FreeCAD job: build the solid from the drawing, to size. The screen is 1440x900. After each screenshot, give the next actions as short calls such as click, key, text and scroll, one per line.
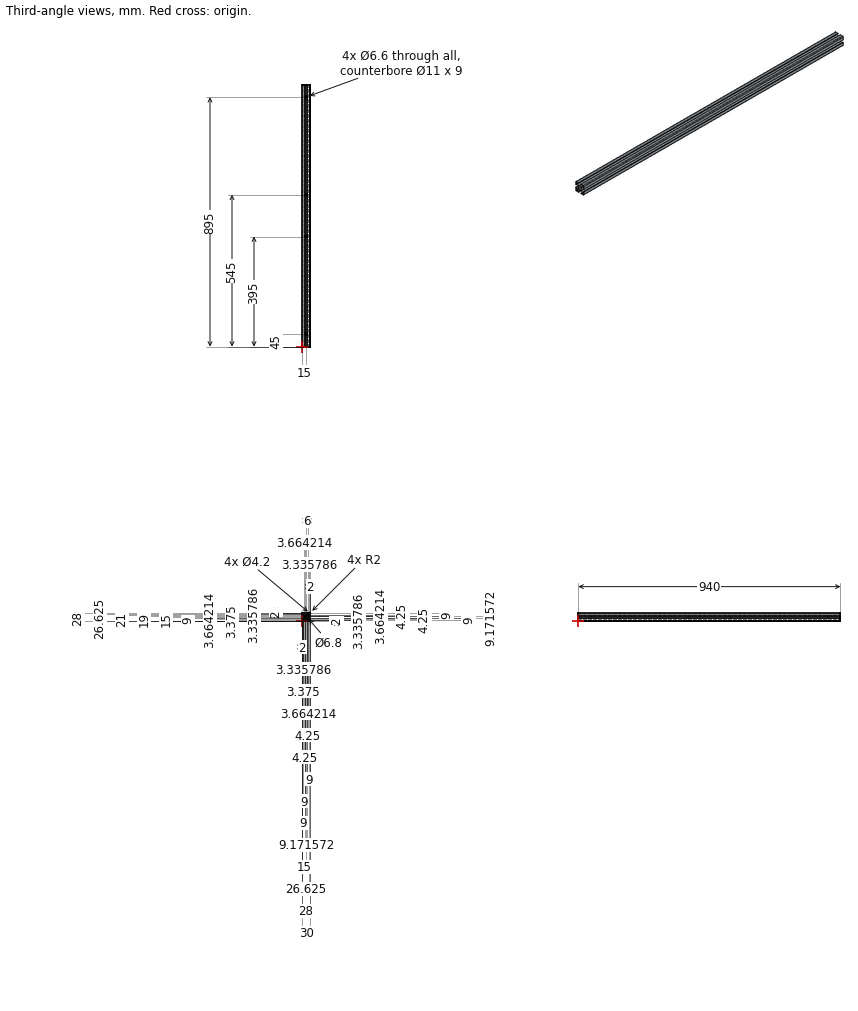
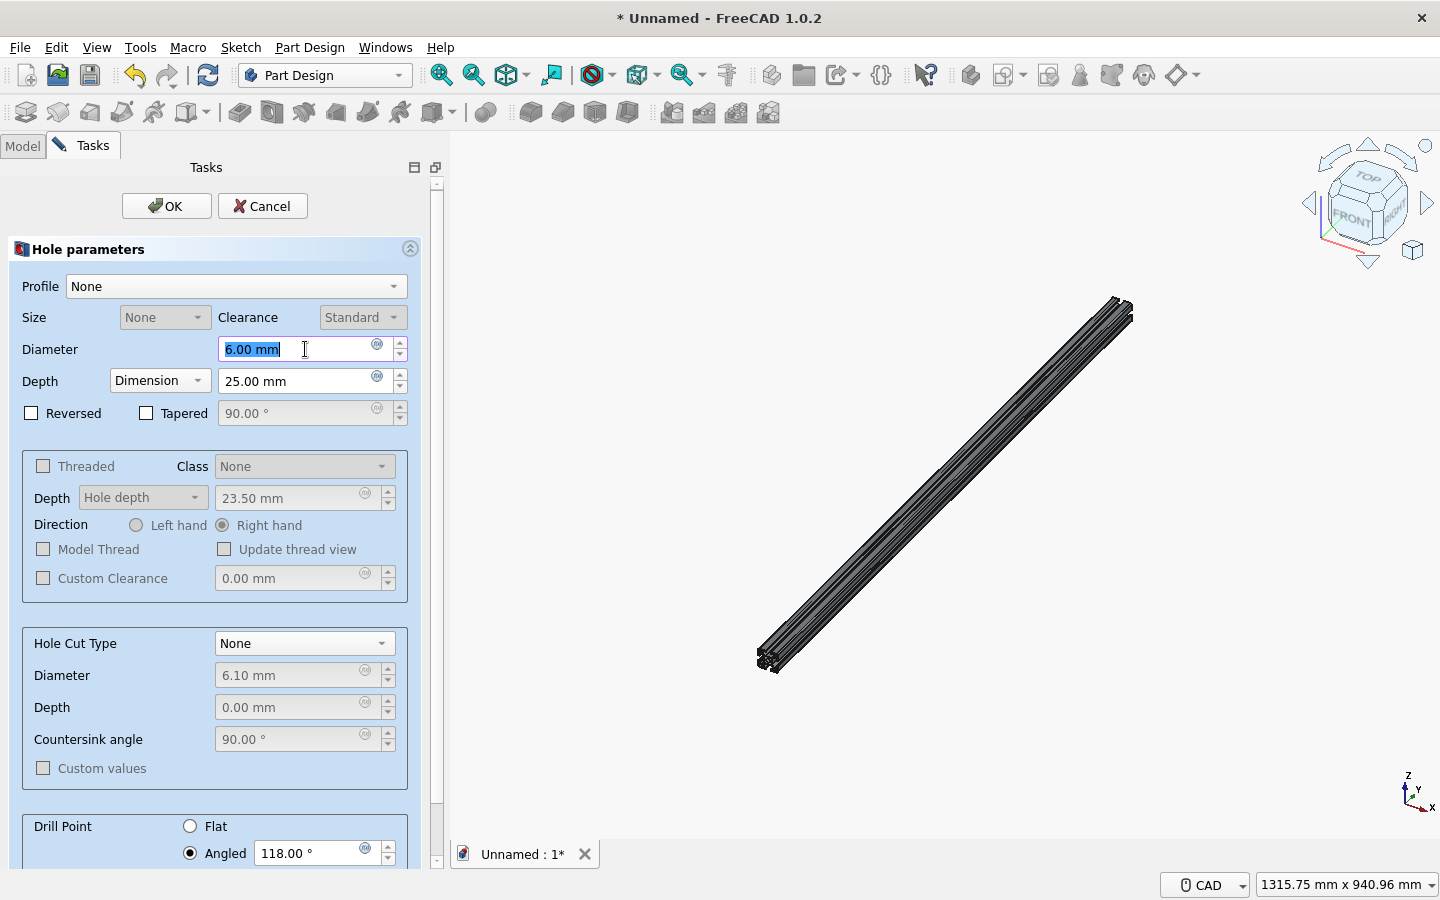
text(6.6)
key(Tab)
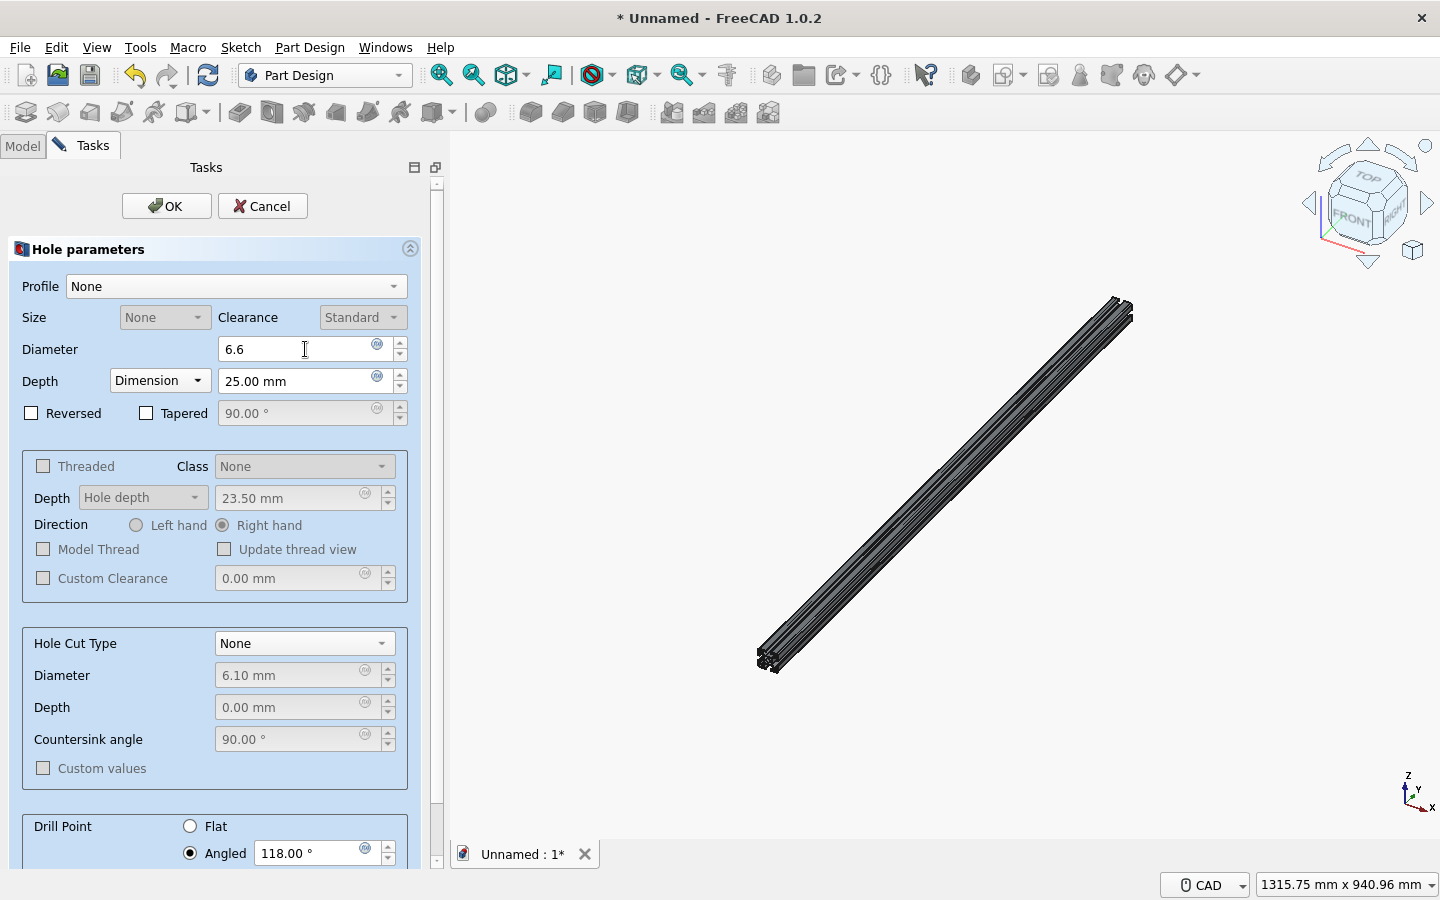
click(161, 380)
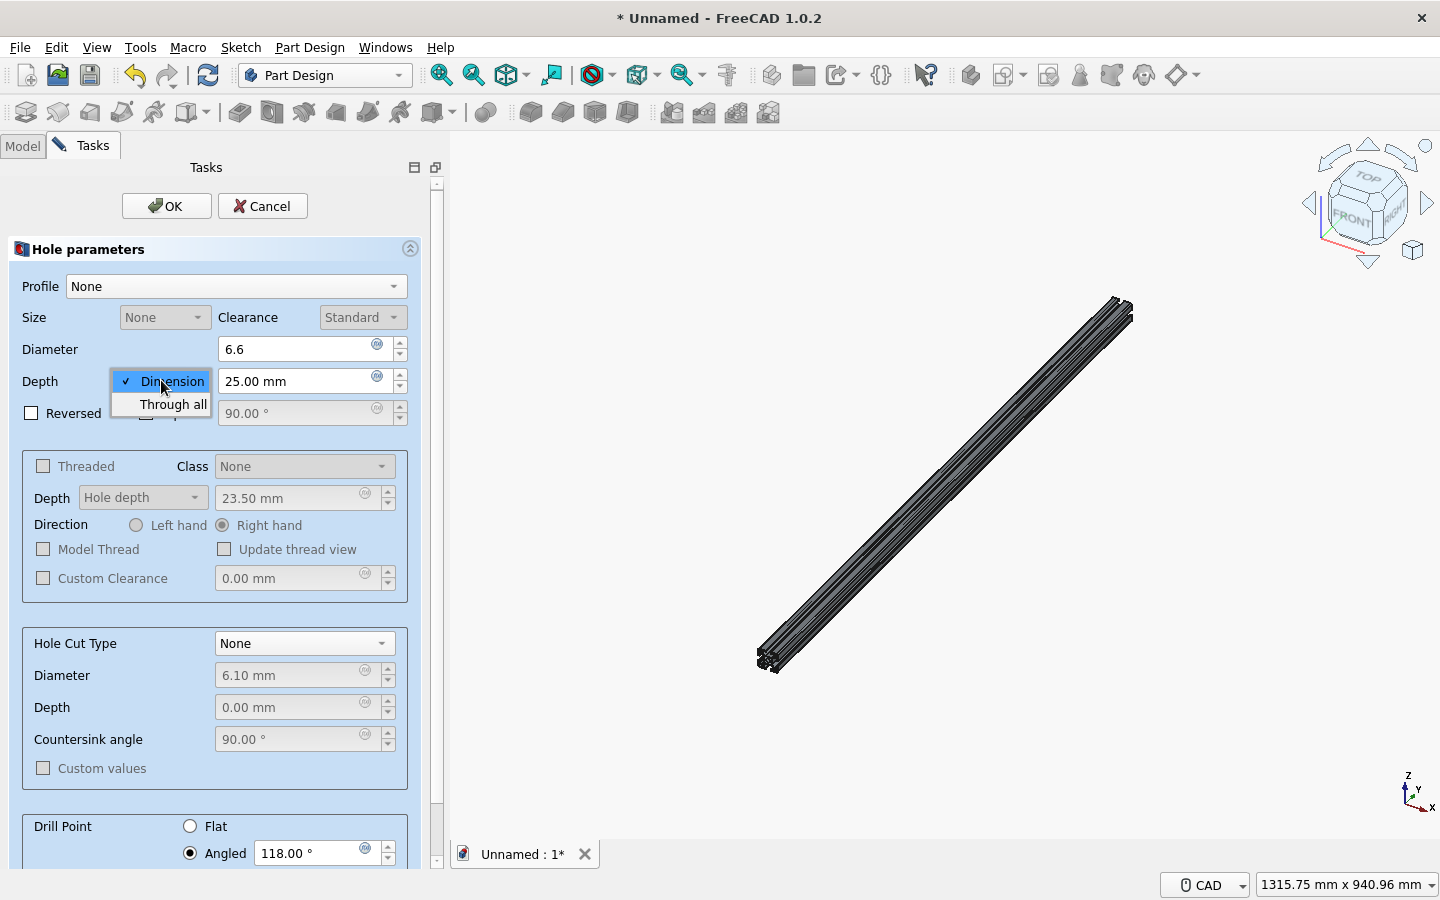
click(160, 404)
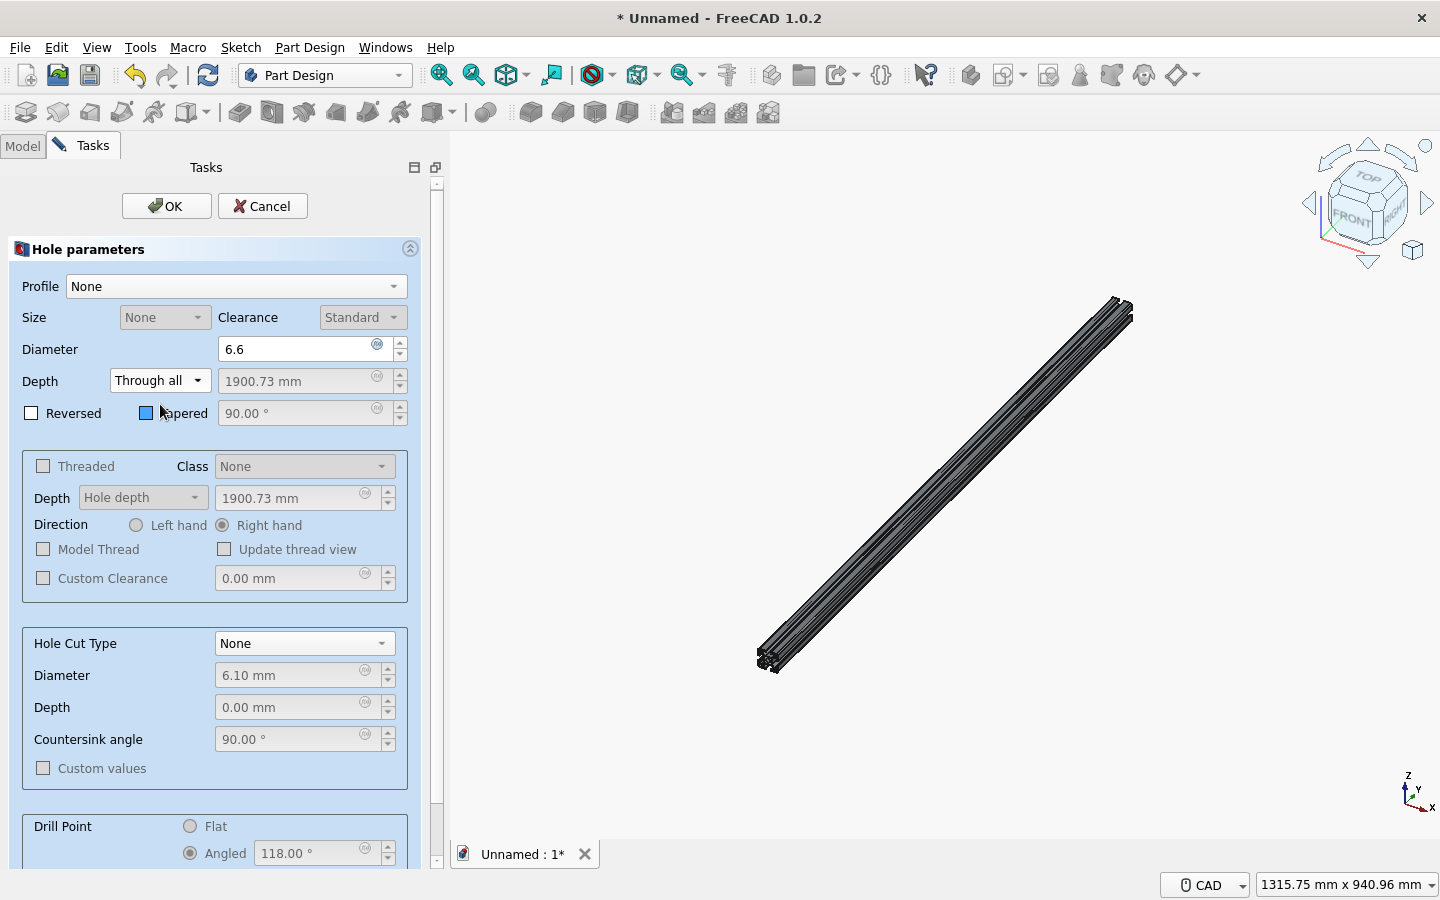
click(30, 413)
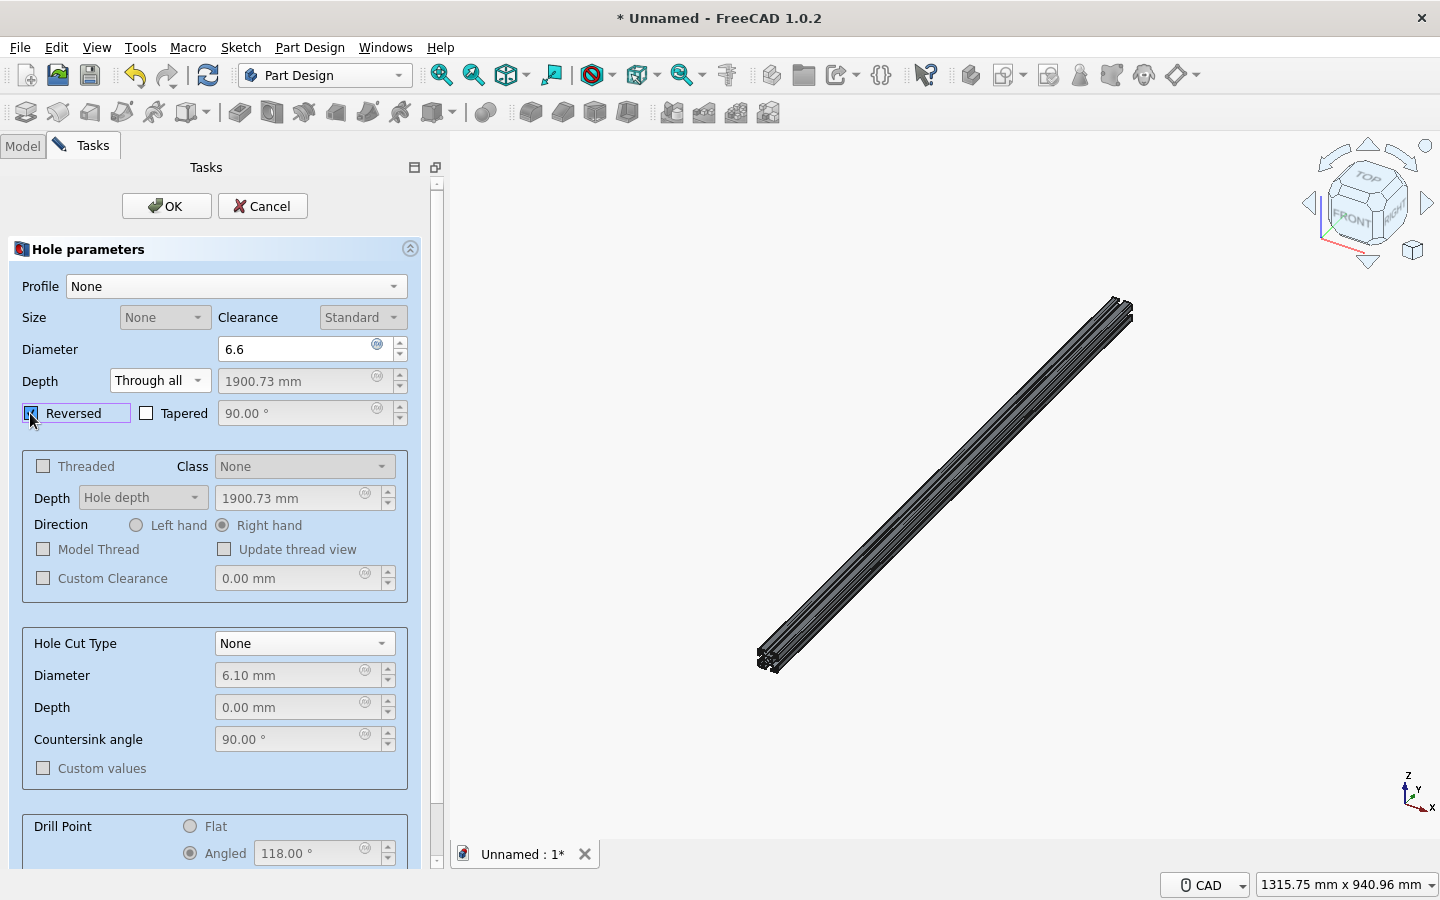
click(306, 644)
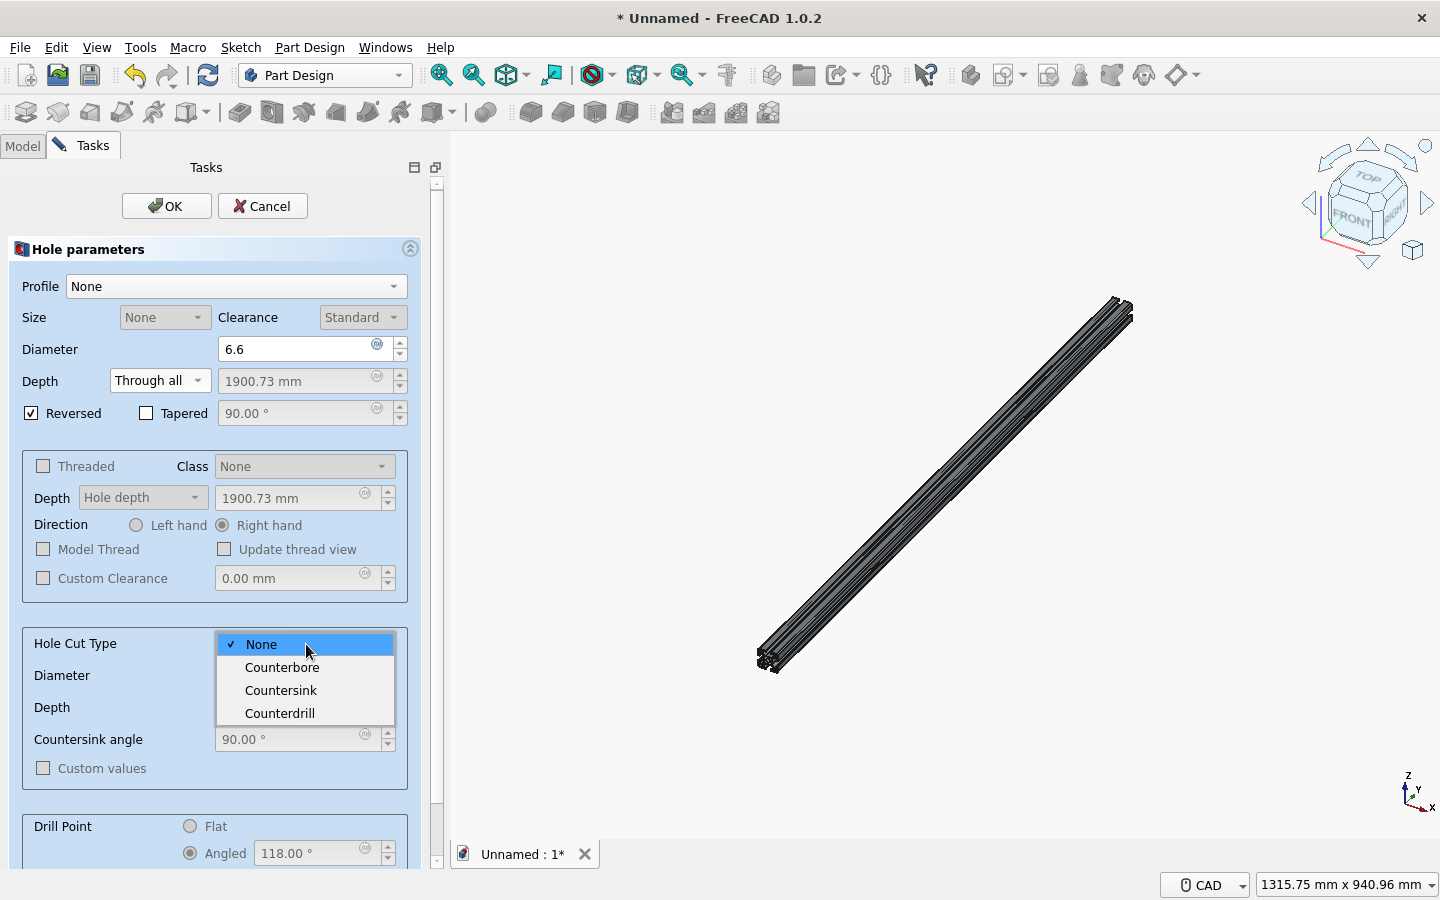
click(304, 668)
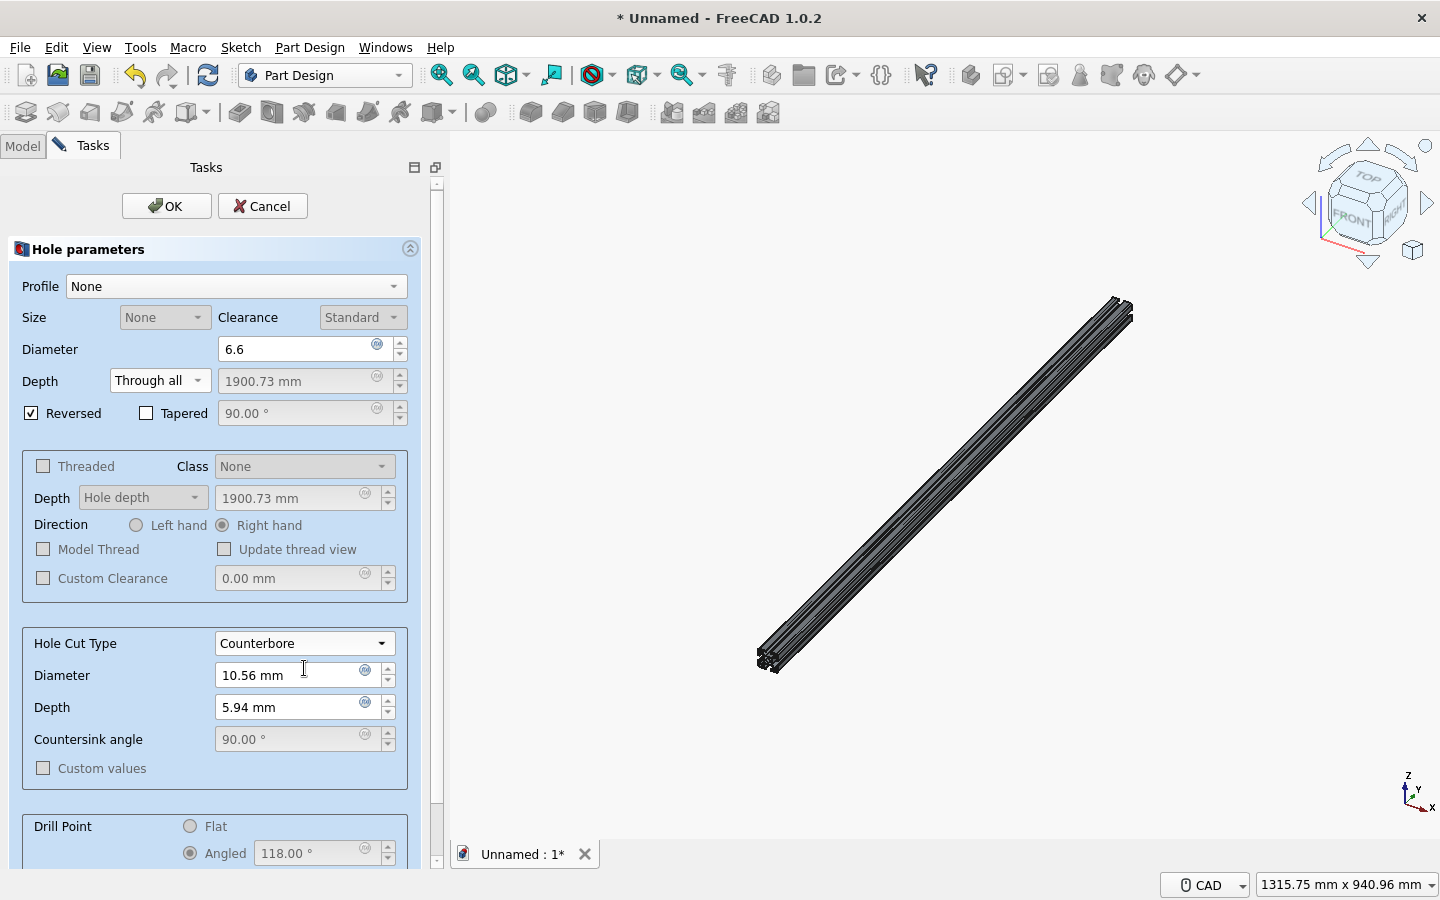
triple_click(298, 675)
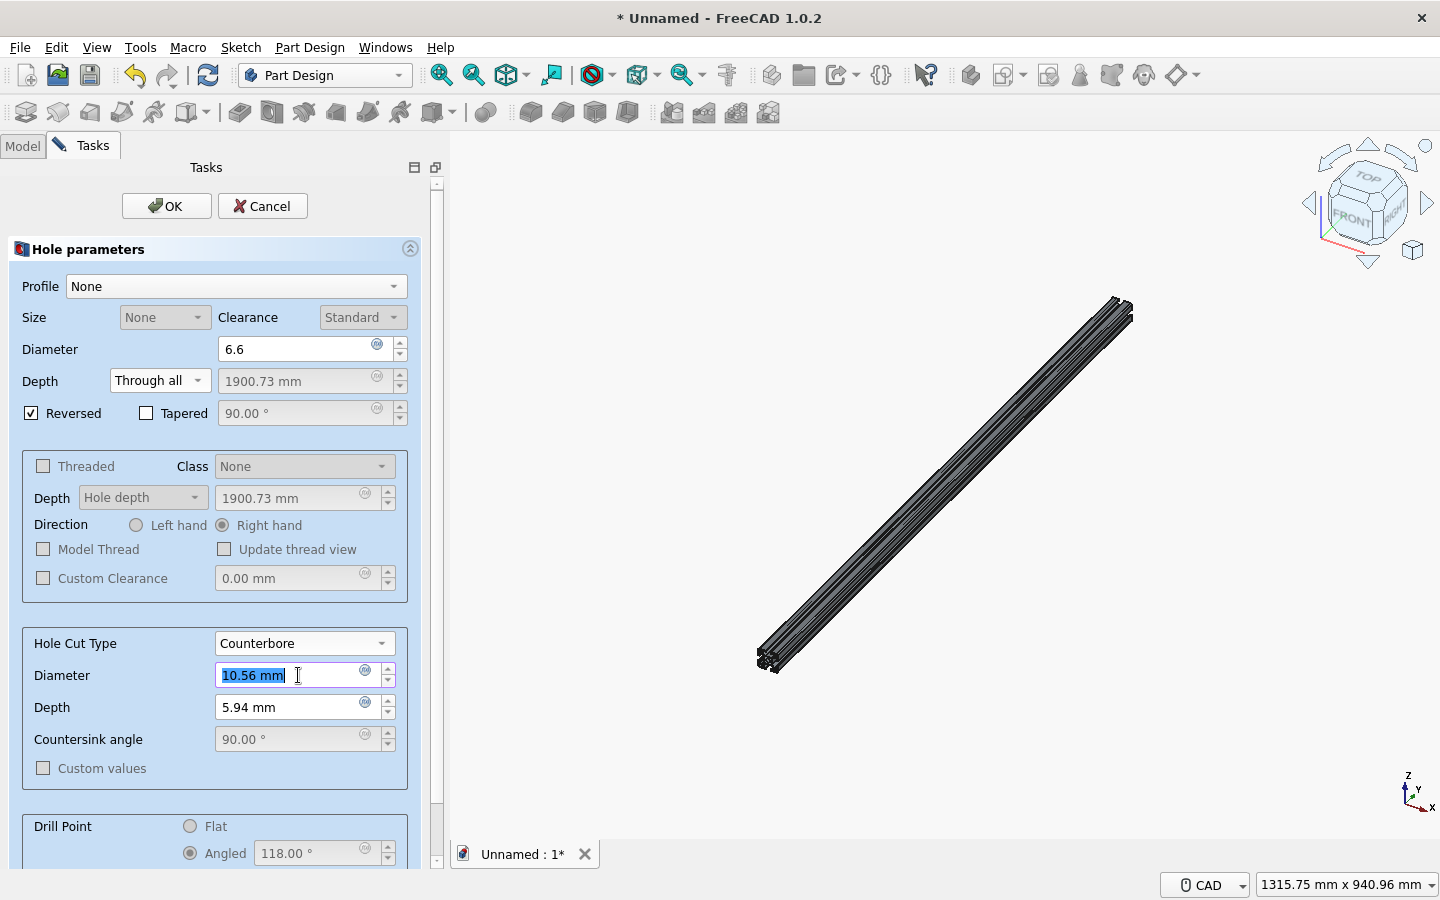
text(11)
key(Tab)